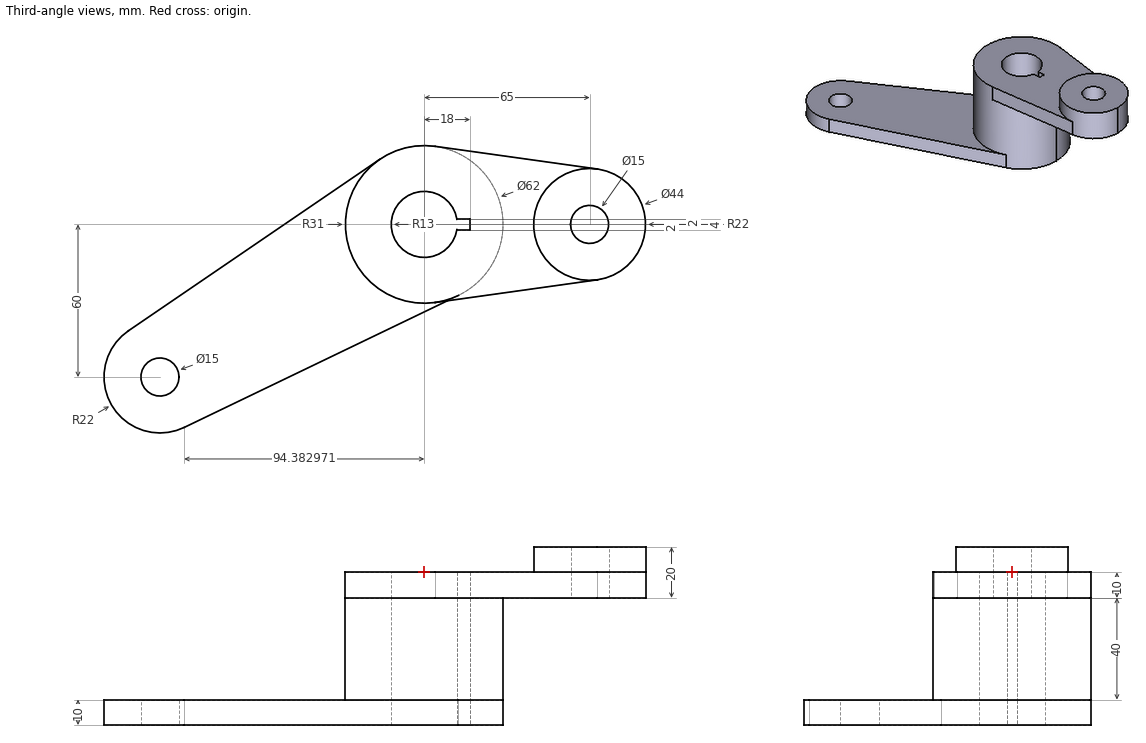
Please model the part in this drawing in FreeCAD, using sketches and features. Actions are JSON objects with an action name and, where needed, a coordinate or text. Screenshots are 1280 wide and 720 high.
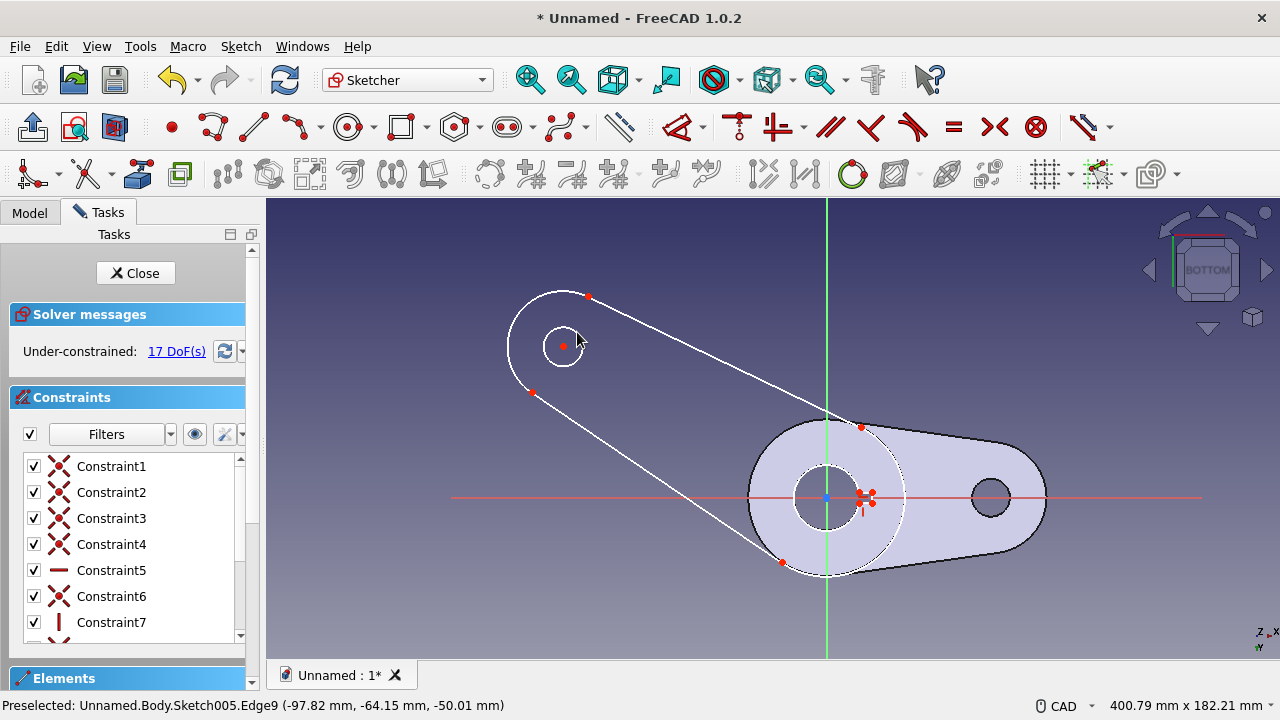
{"action": "left_click", "coordinate": [707, 512]}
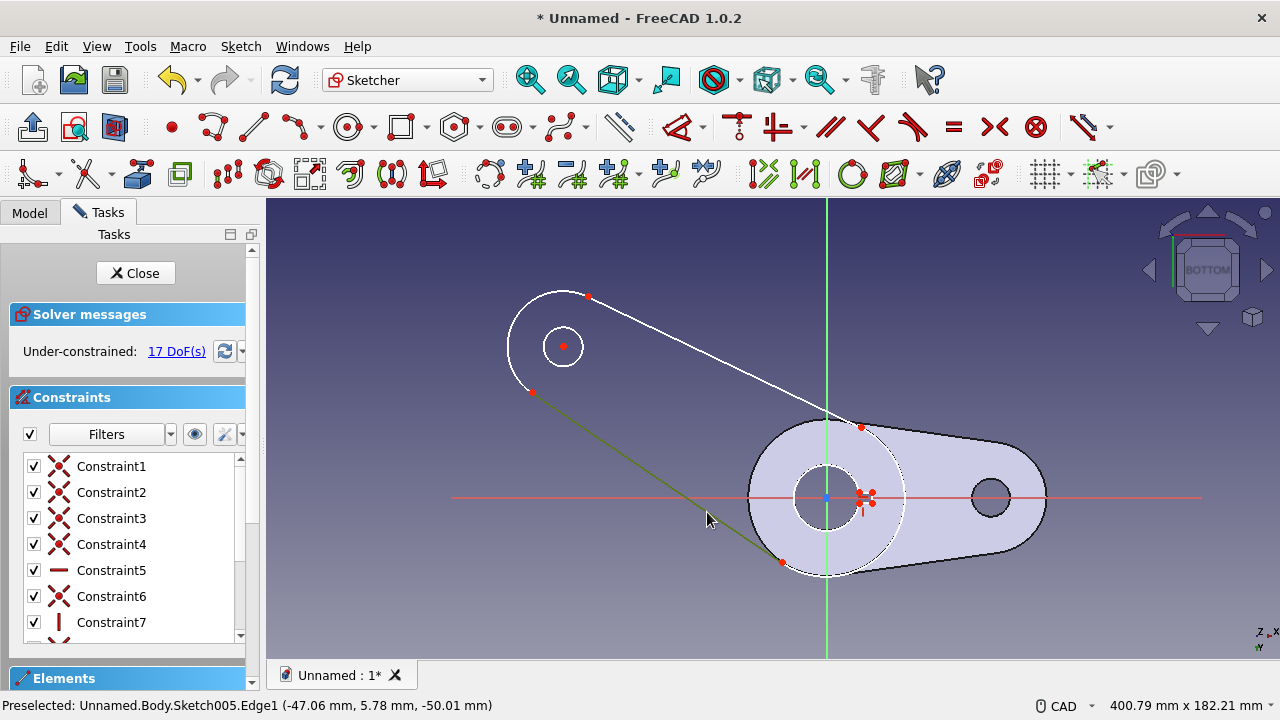
{"action": "left_click", "coordinate": [539, 297]}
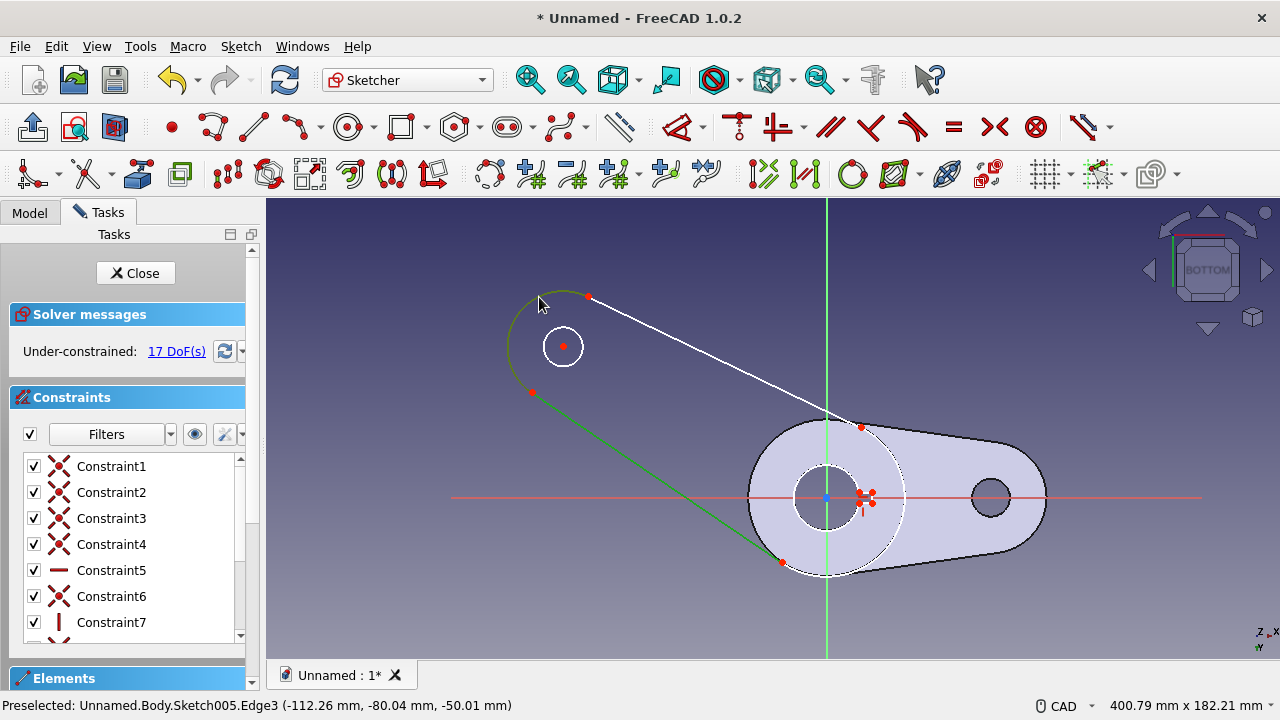
{"action": "key", "text": "t"}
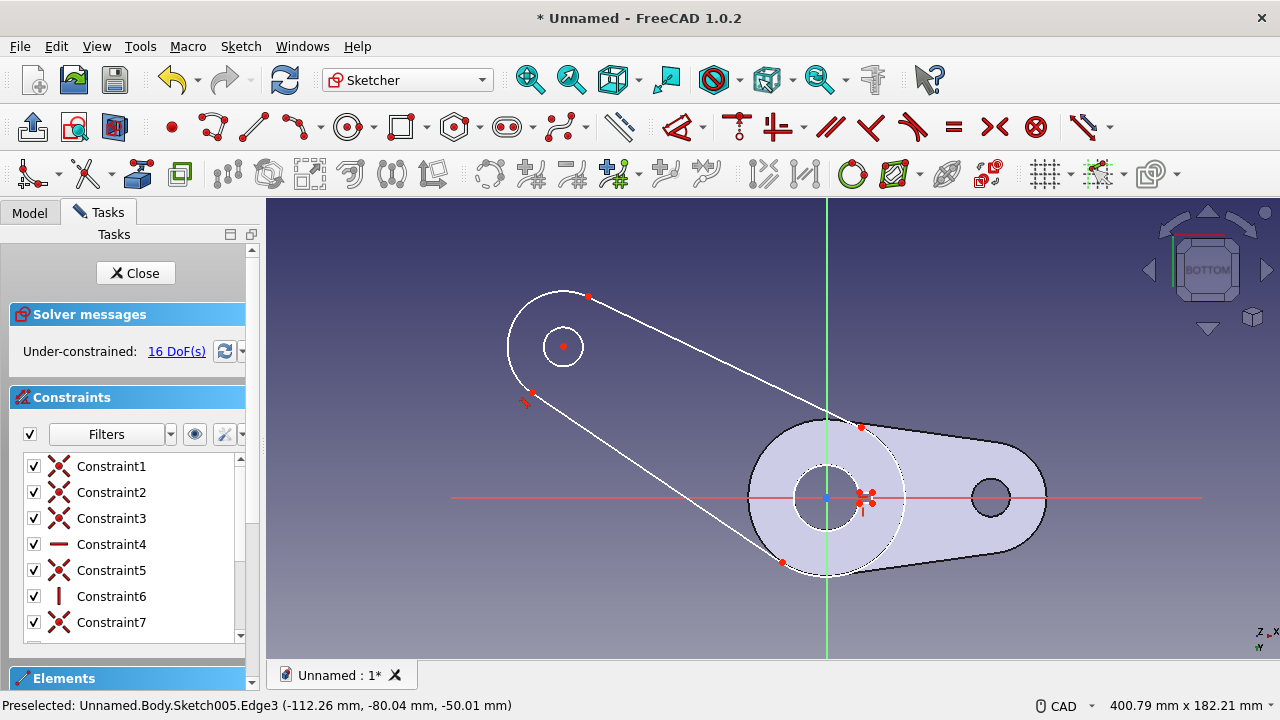
{"action": "left_click", "coordinate": [707, 512]}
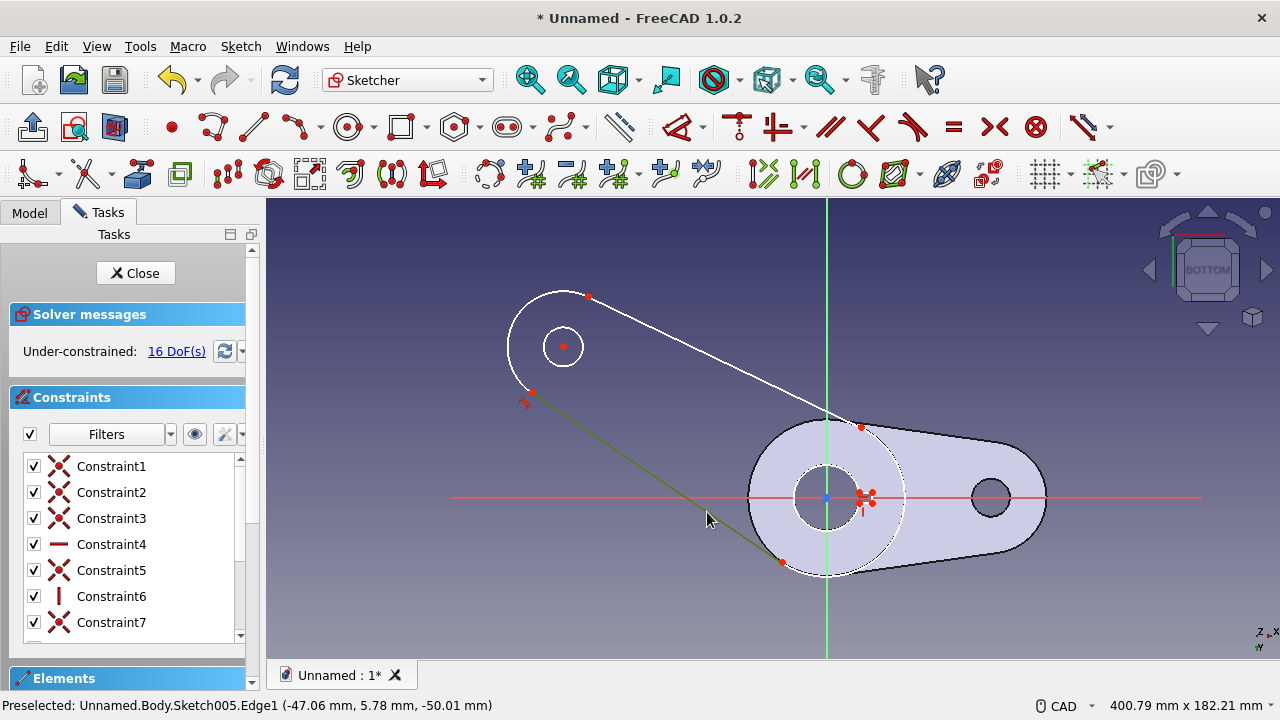
{"action": "left_click", "coordinate": [856, 571]}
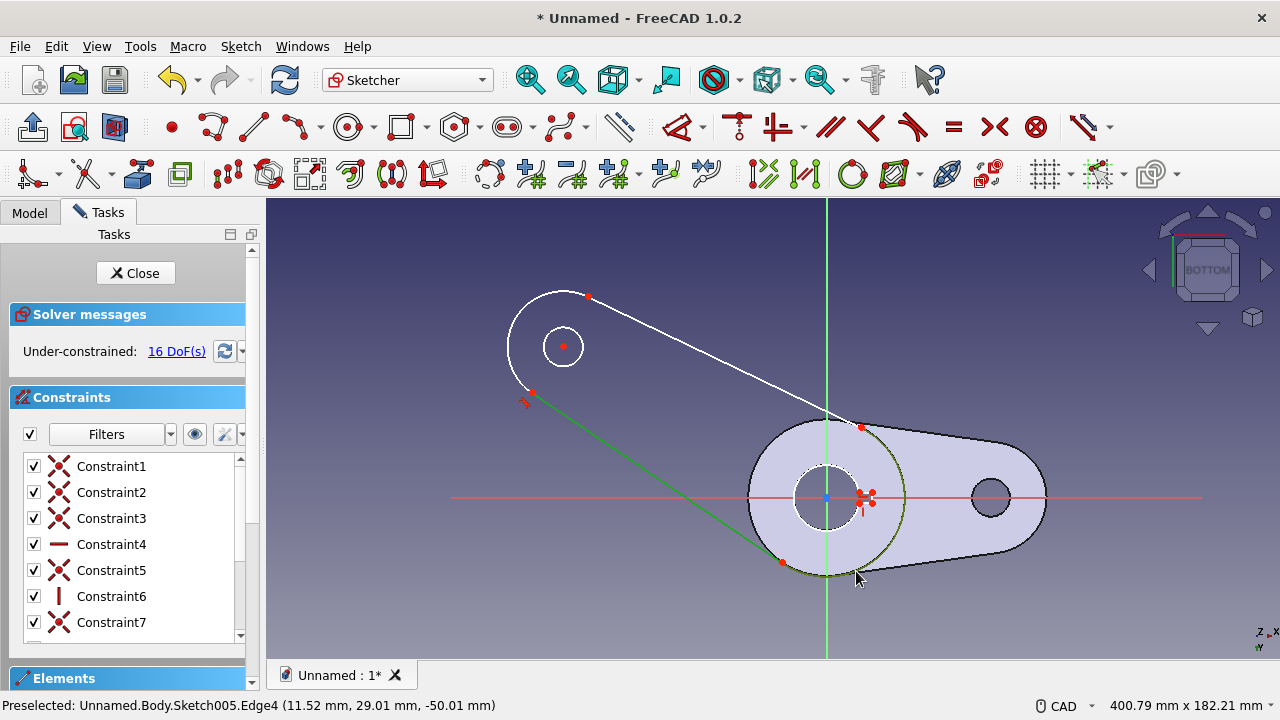
{"action": "left_click", "coordinate": [913, 128]}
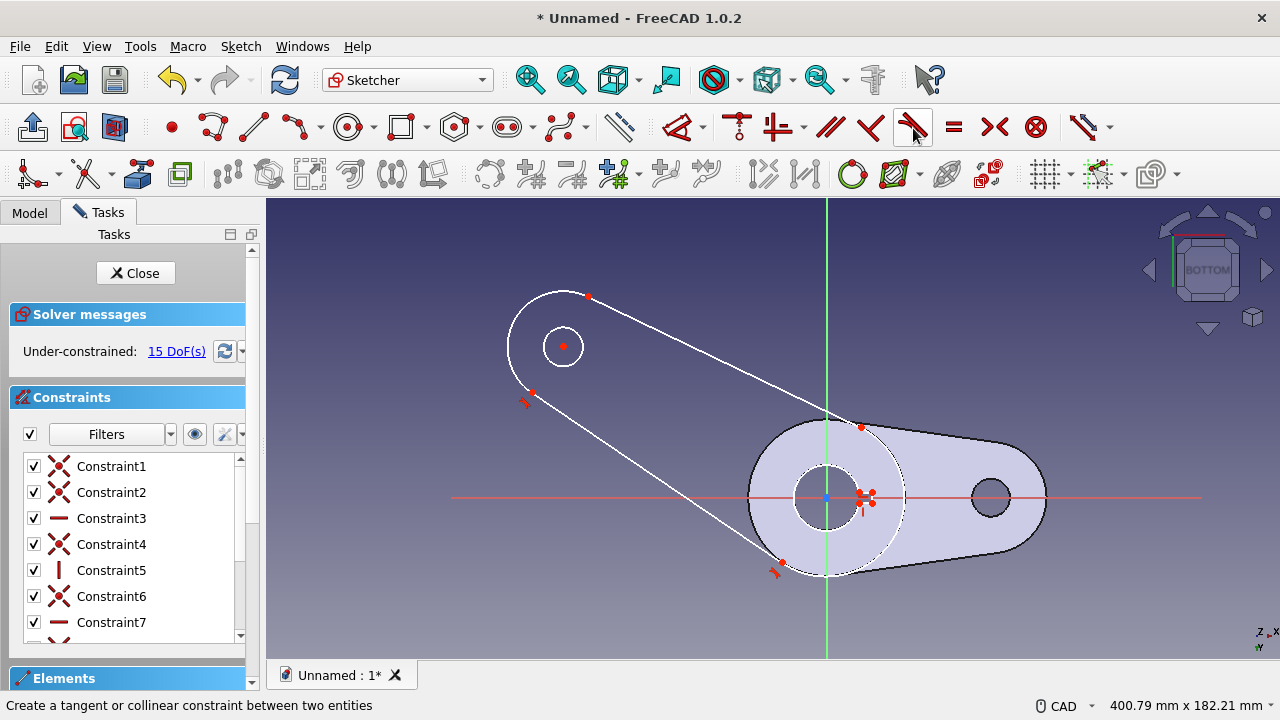
{"action": "left_click", "coordinate": [670, 336]}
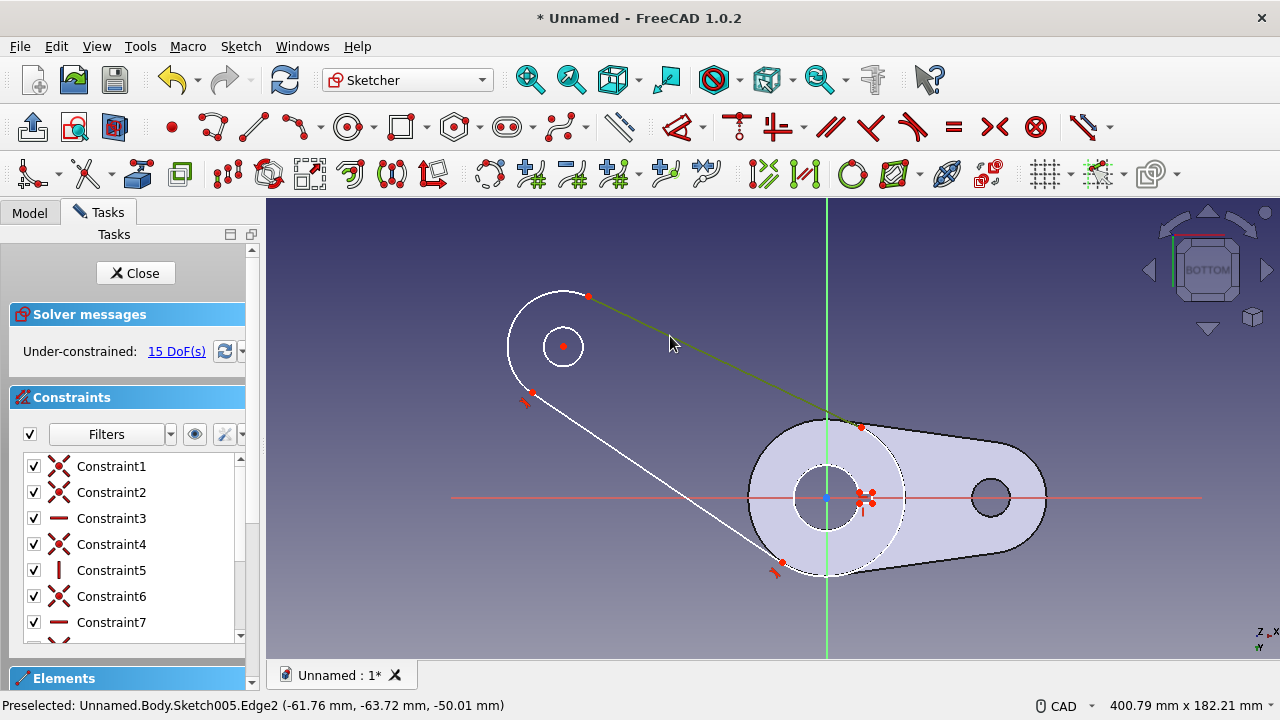
{"action": "left_click", "coordinate": [539, 297]}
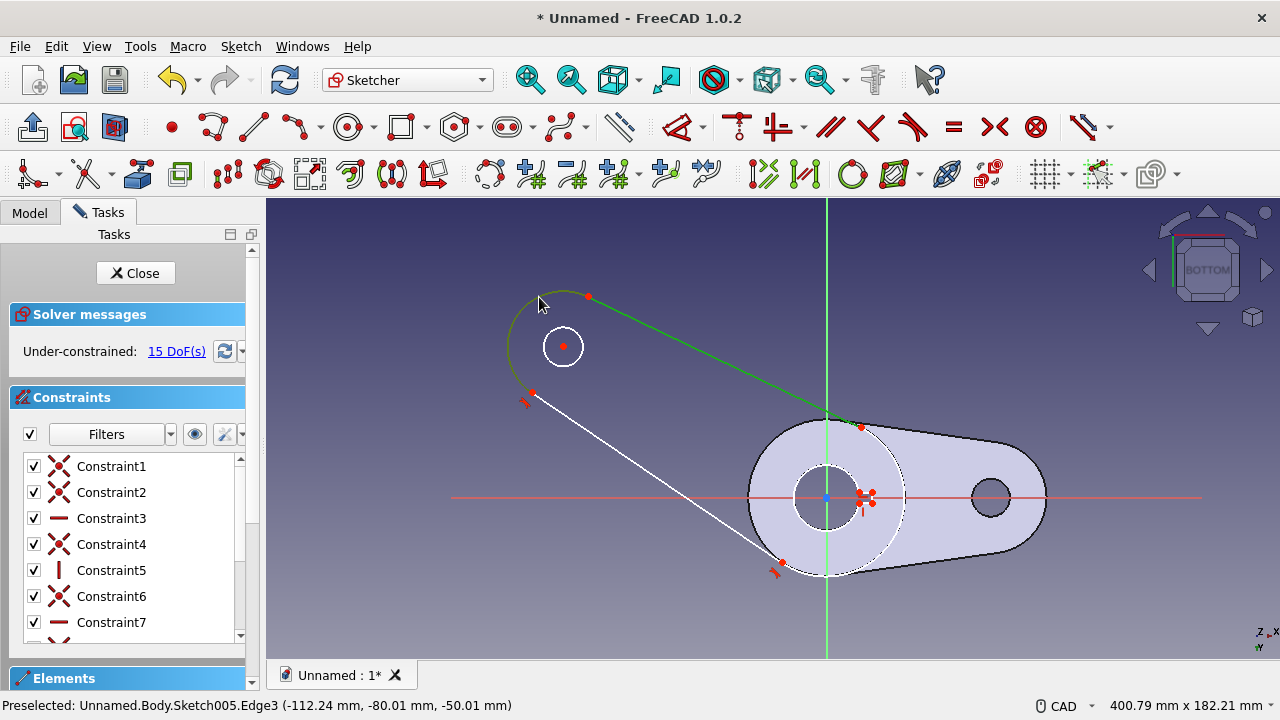
{"action": "key", "text": "t"}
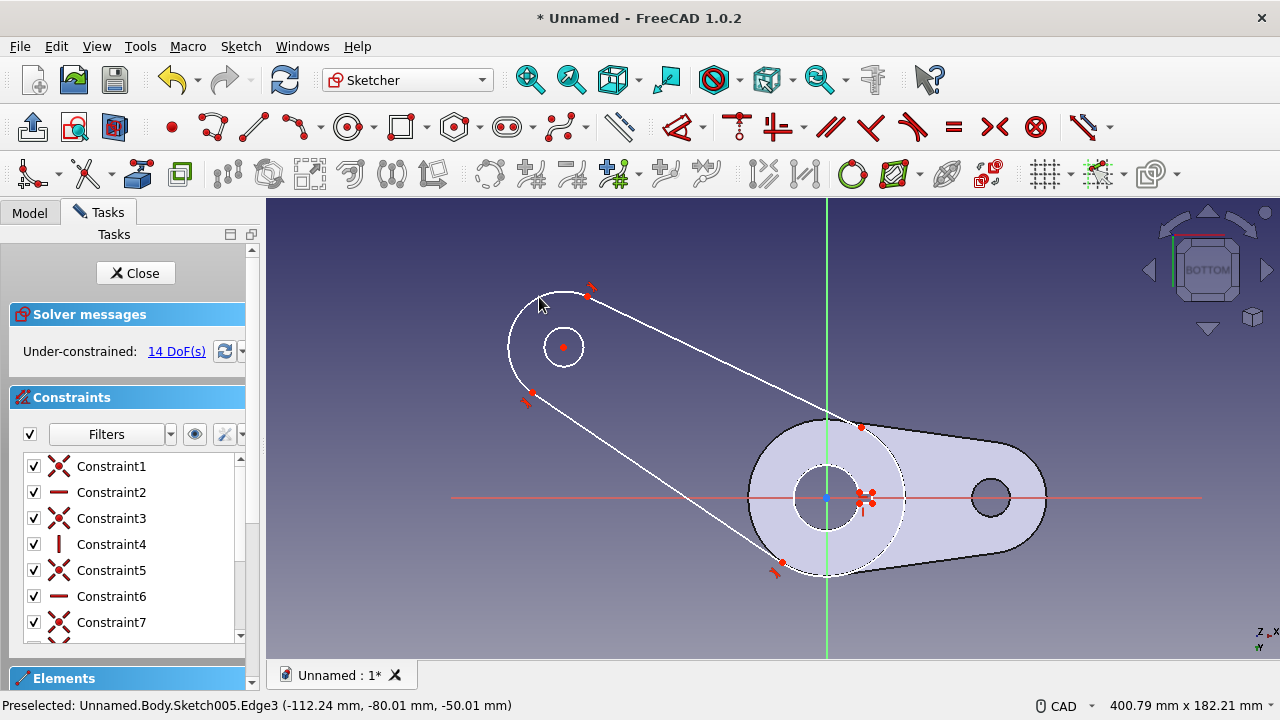
{"action": "left_click", "coordinate": [670, 336]}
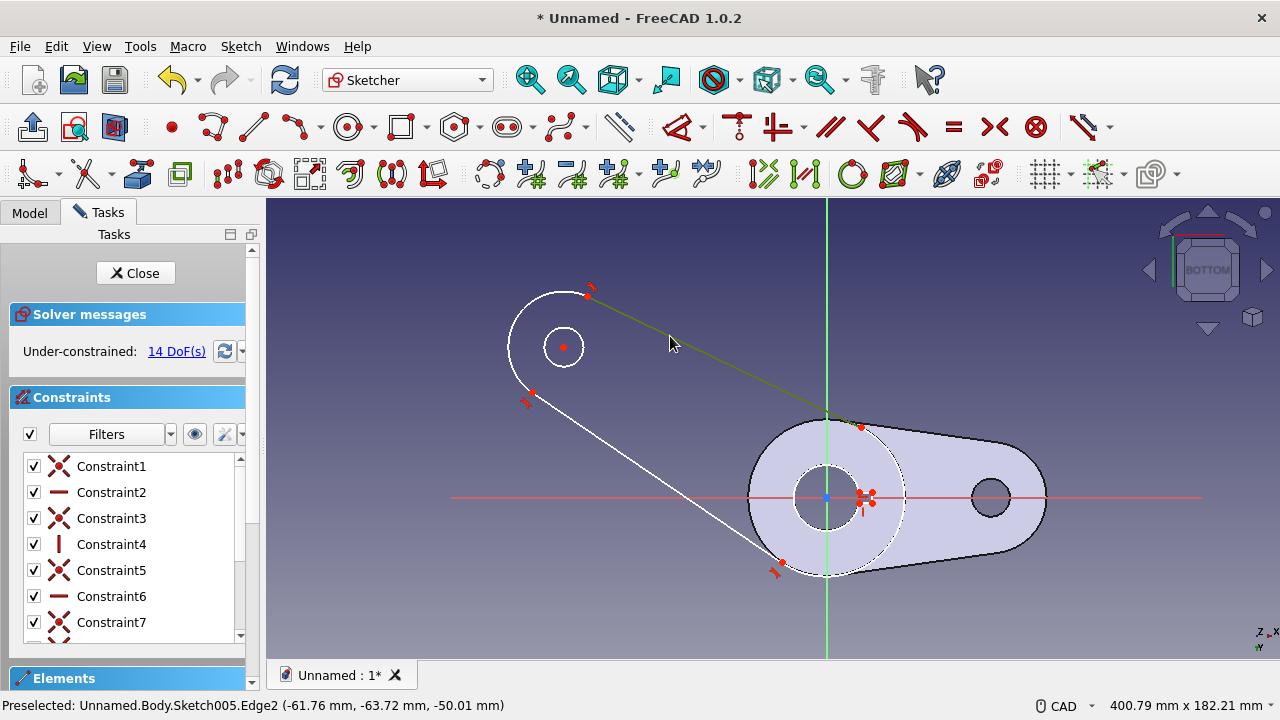
{"action": "left_click", "coordinate": [856, 571]}